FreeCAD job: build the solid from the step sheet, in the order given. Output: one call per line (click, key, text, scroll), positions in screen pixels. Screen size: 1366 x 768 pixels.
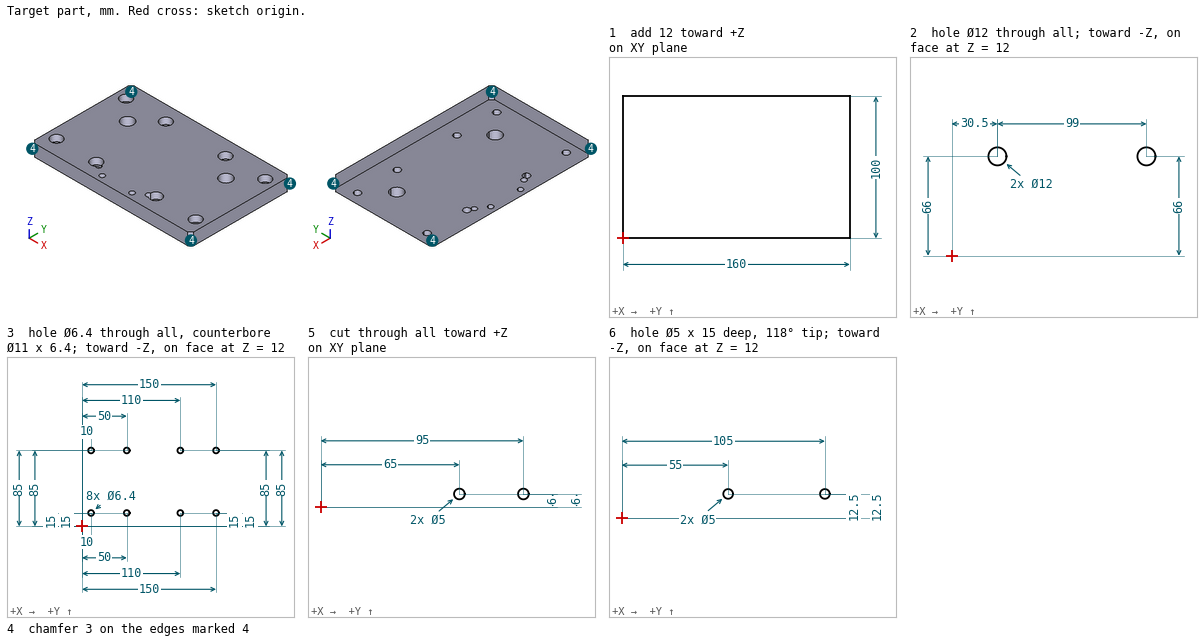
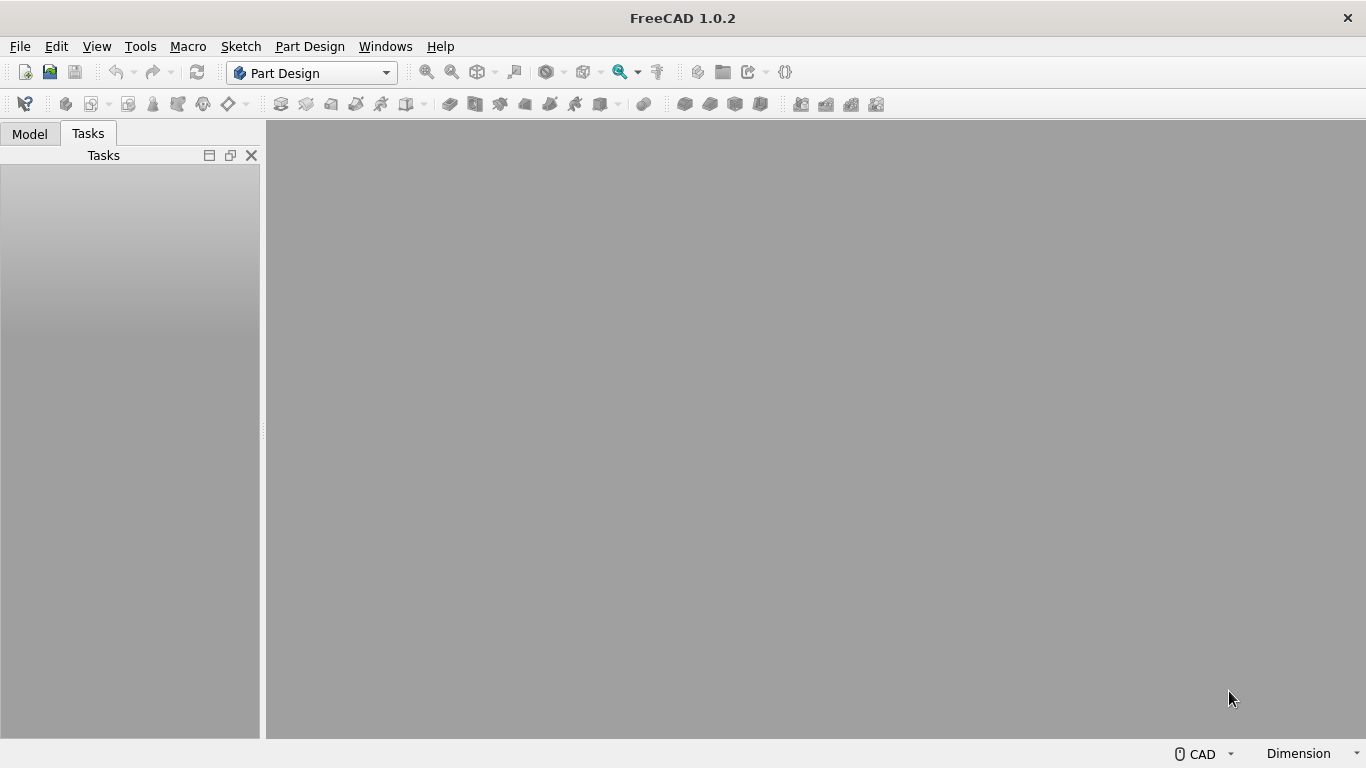
click(25, 72)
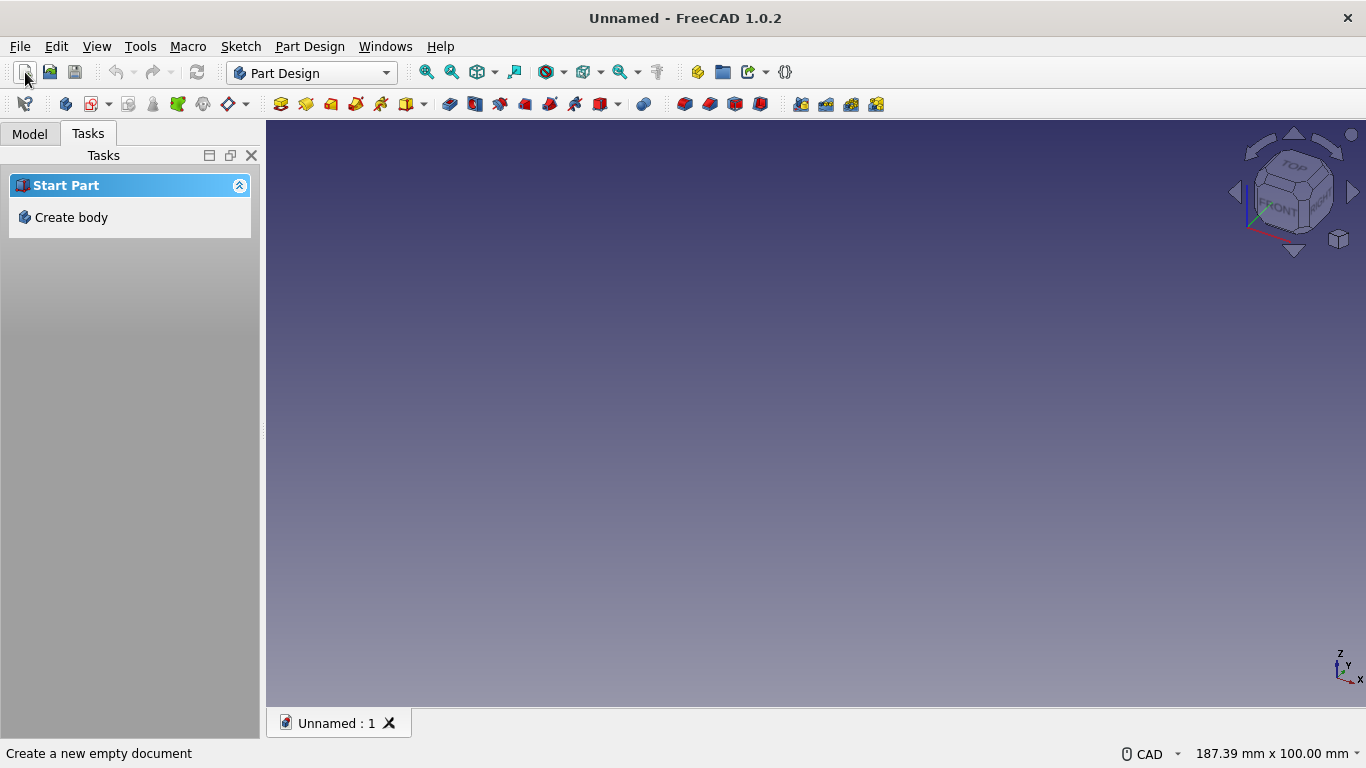
click(90, 104)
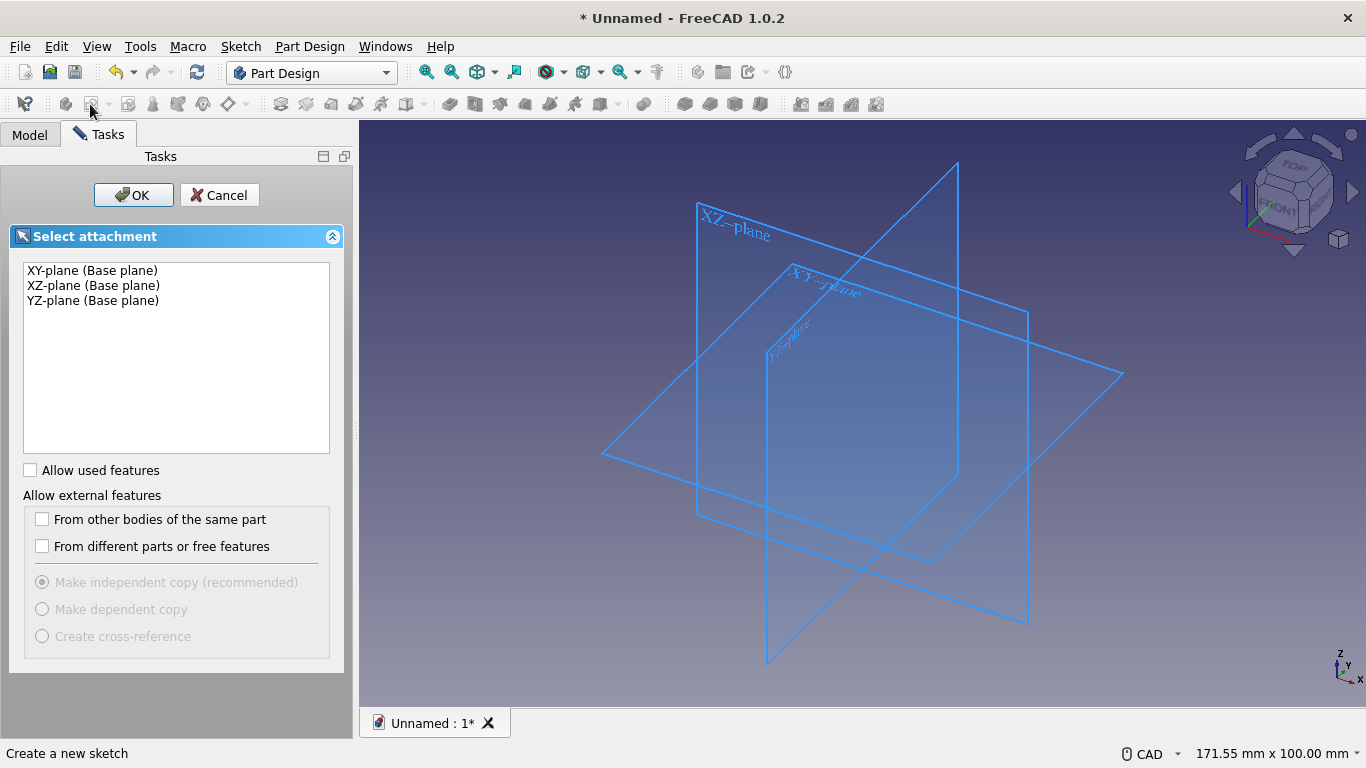
click(84, 270)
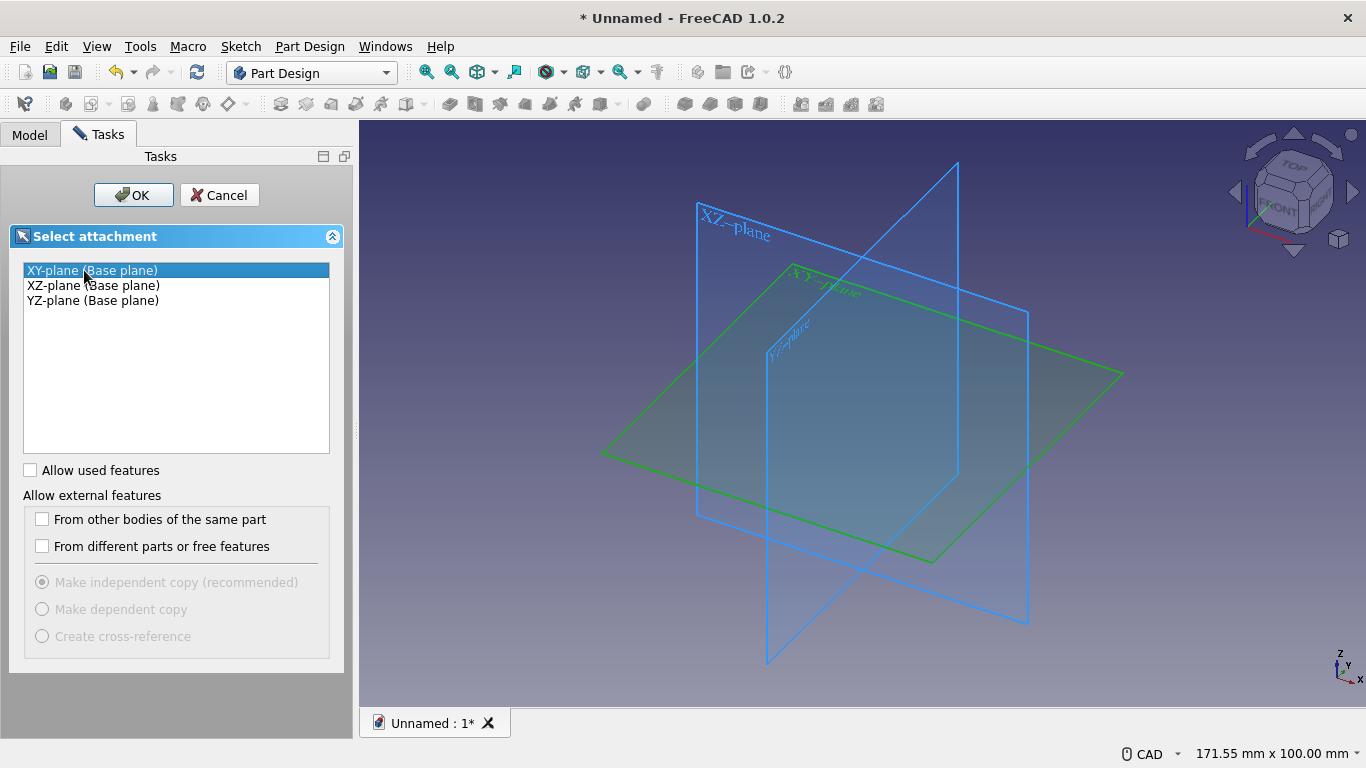
click(134, 195)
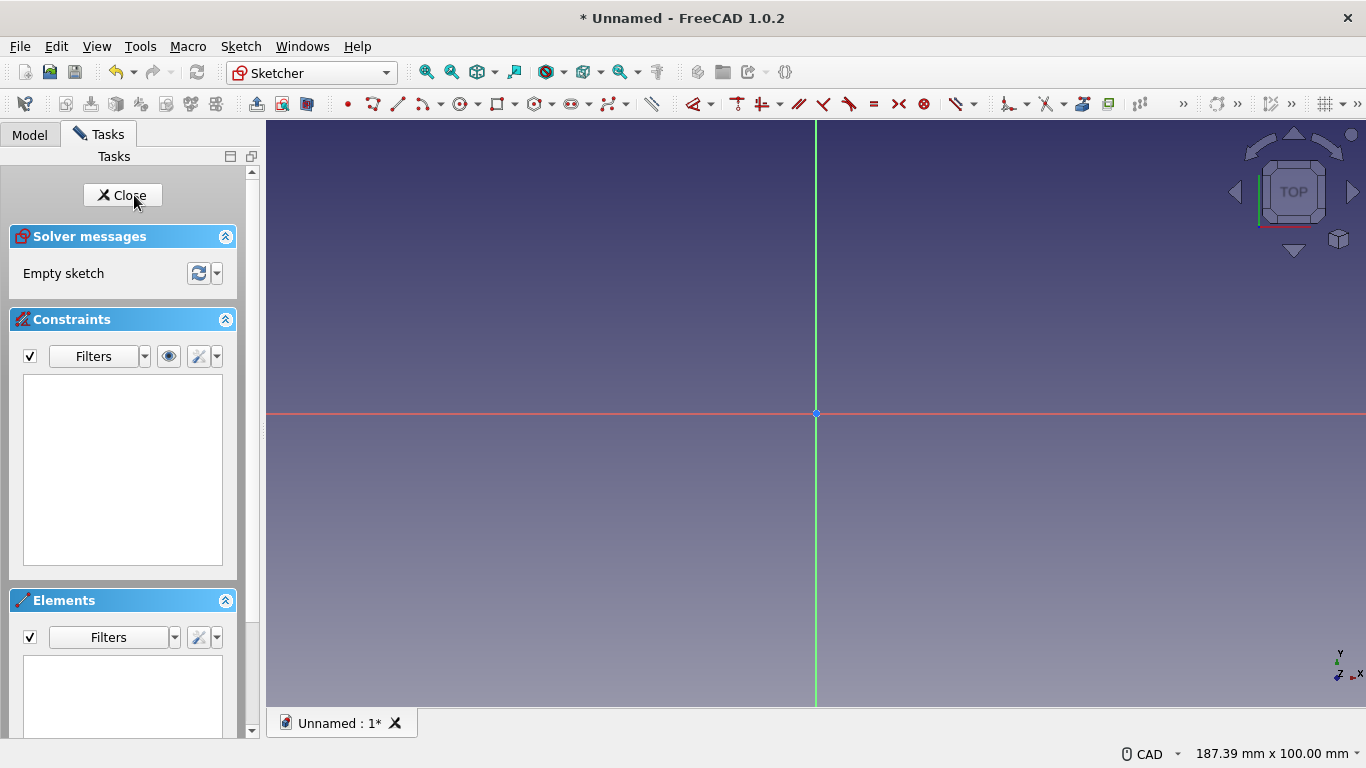
scroll(294, 679, down, 3)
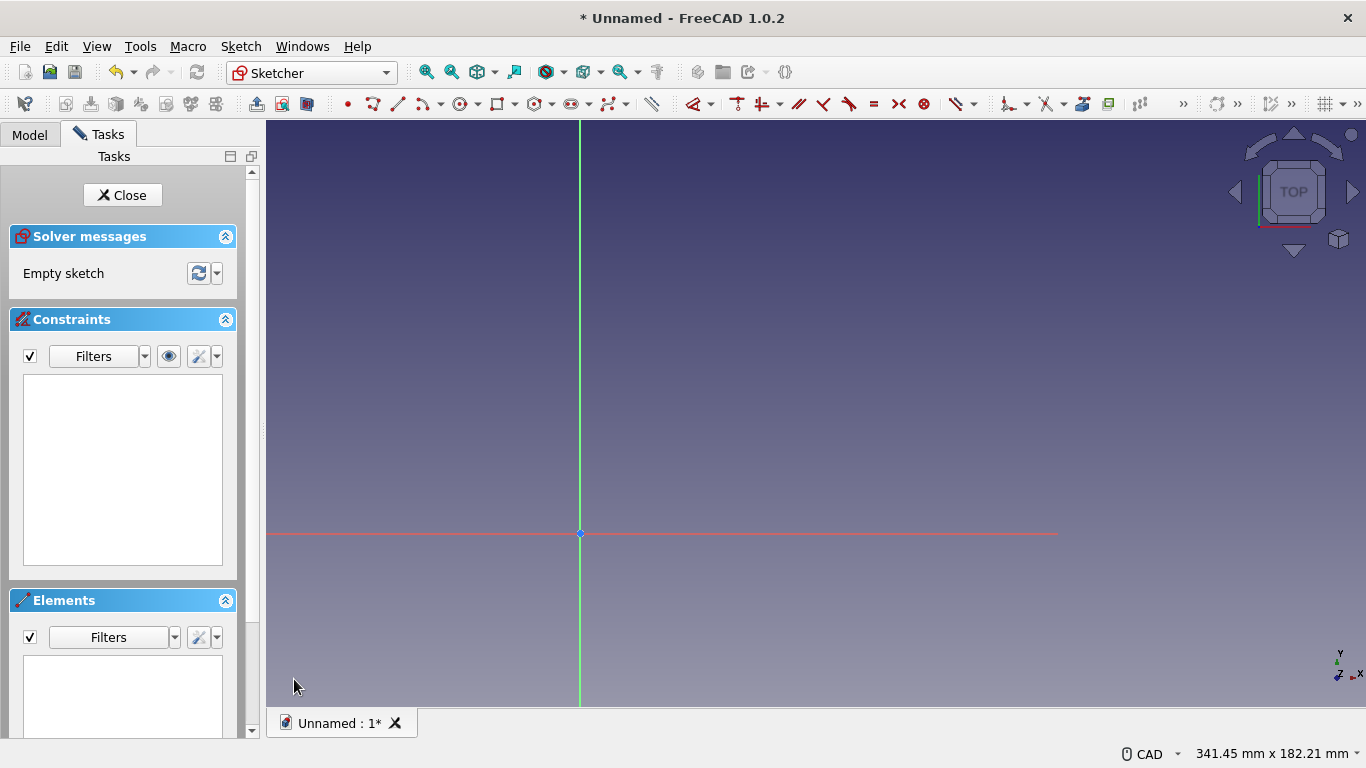
click(496, 104)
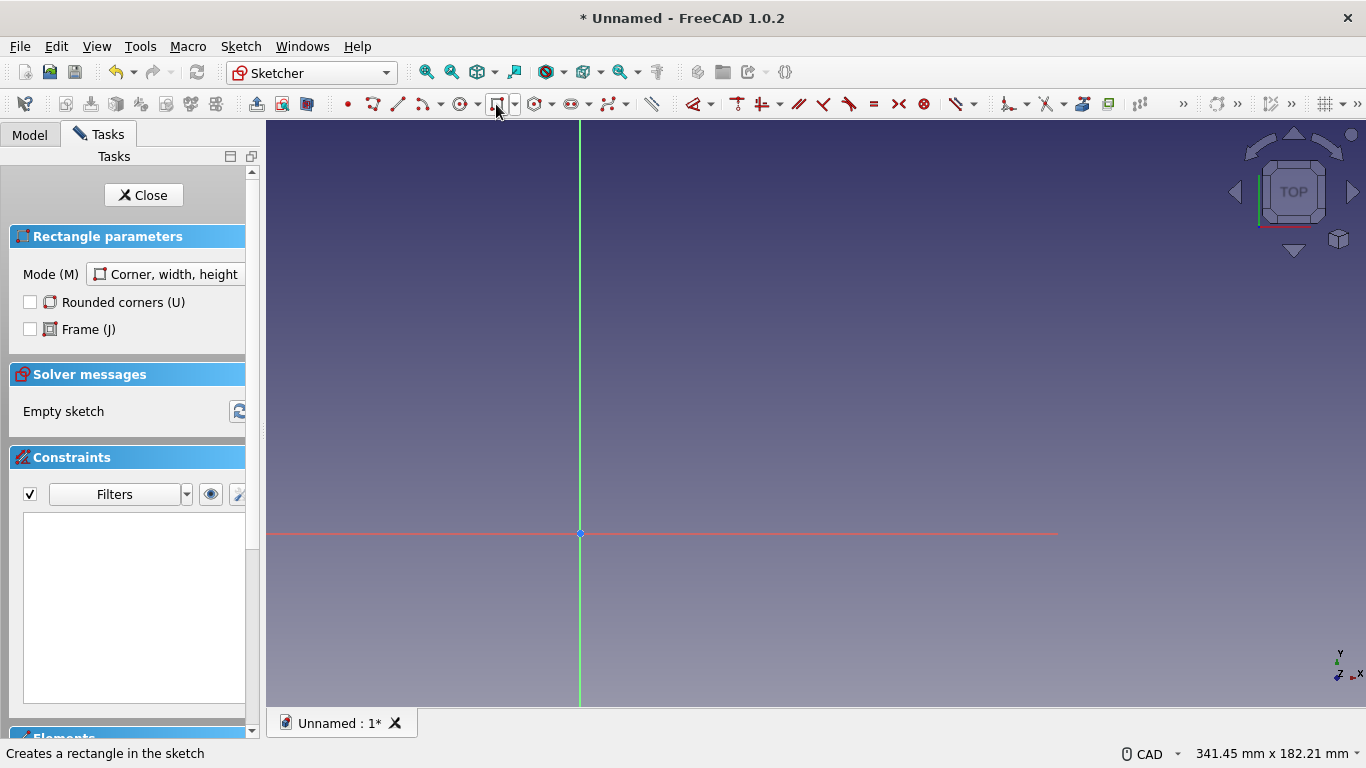
click(580, 534)
click(1096, 212)
key(Escape)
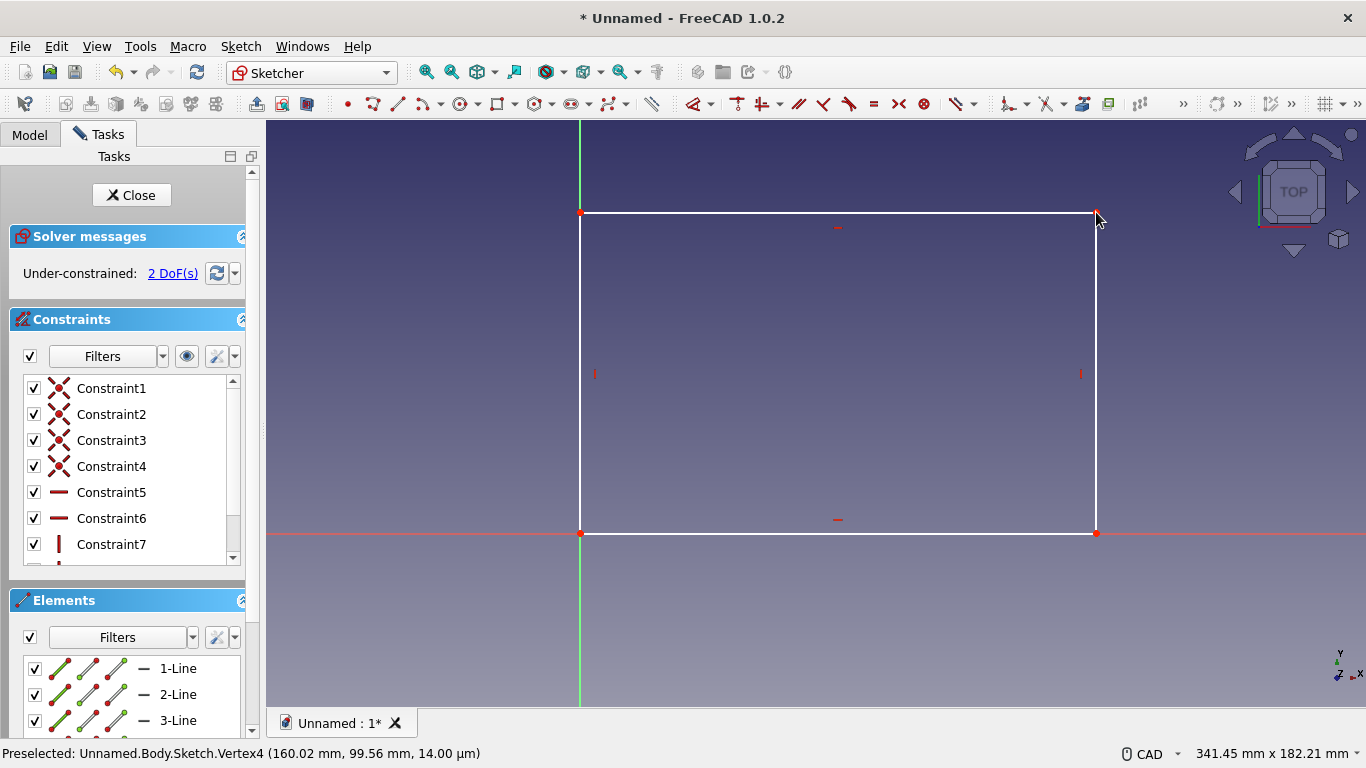
click(735, 534)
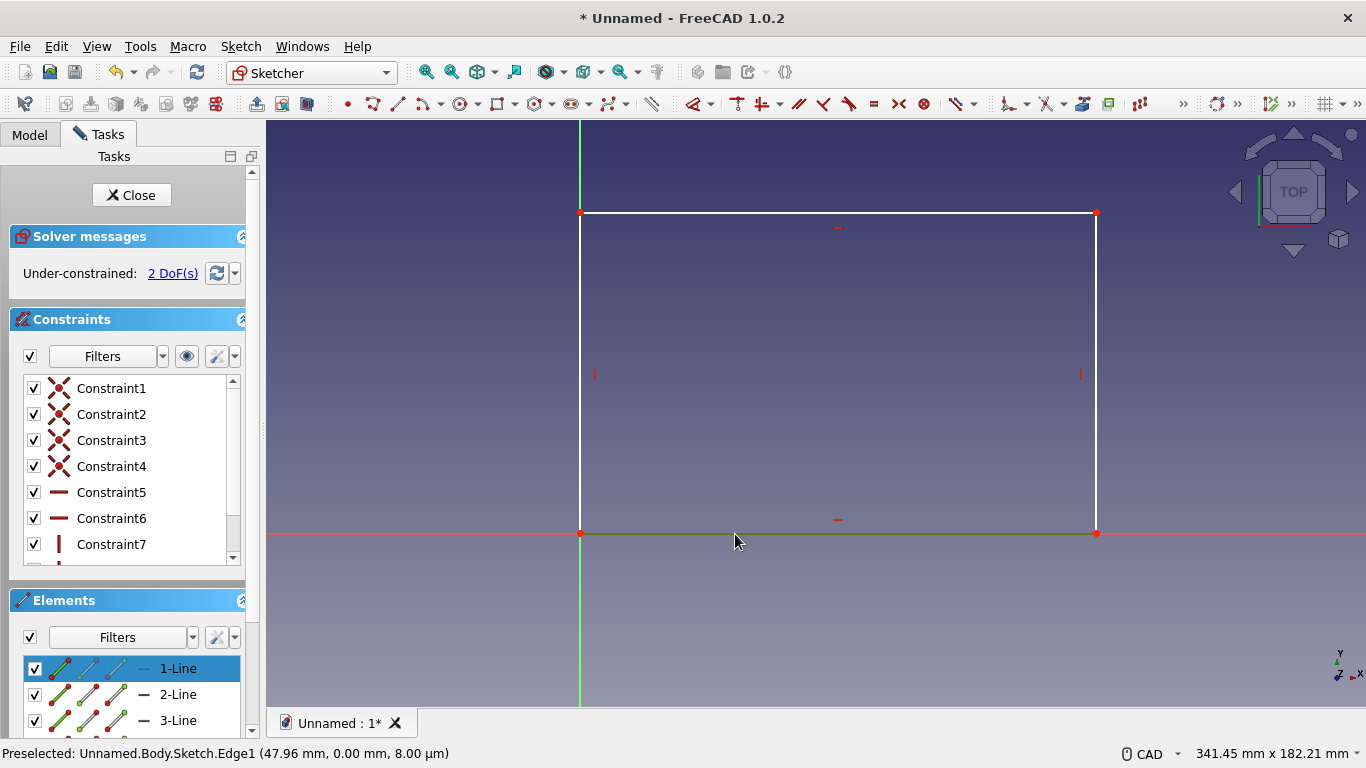
key(l)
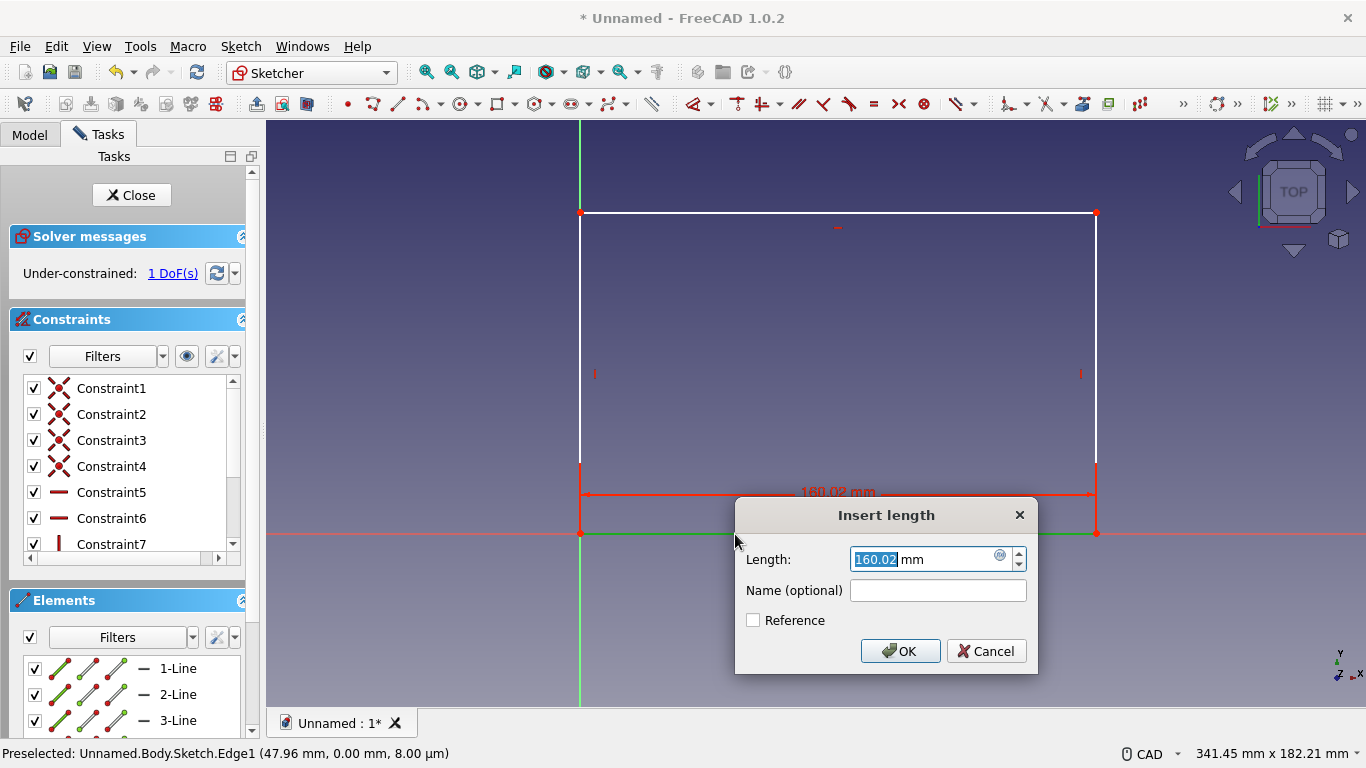
text(160)
key(Return)